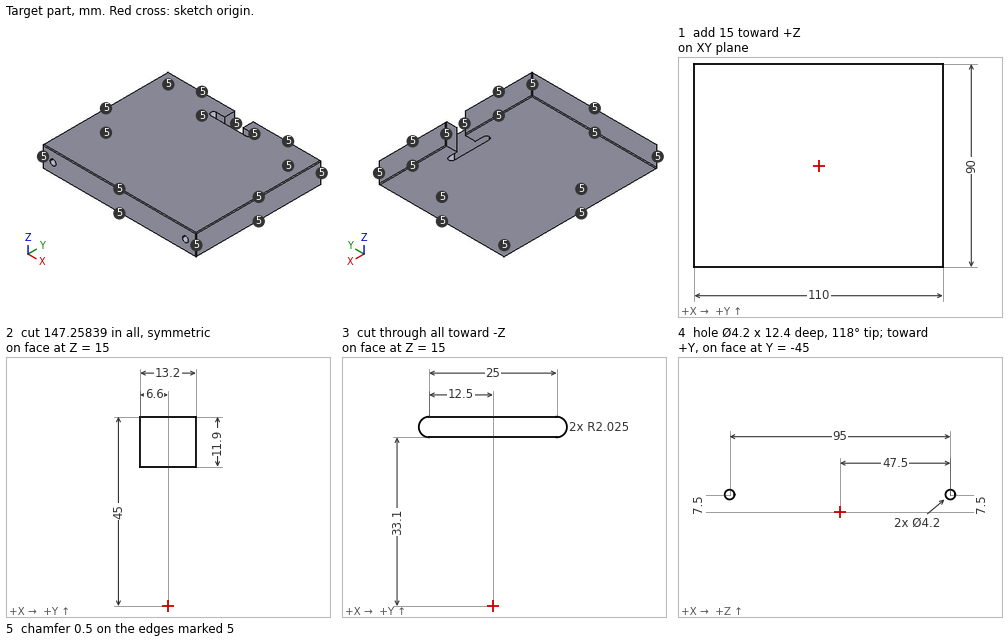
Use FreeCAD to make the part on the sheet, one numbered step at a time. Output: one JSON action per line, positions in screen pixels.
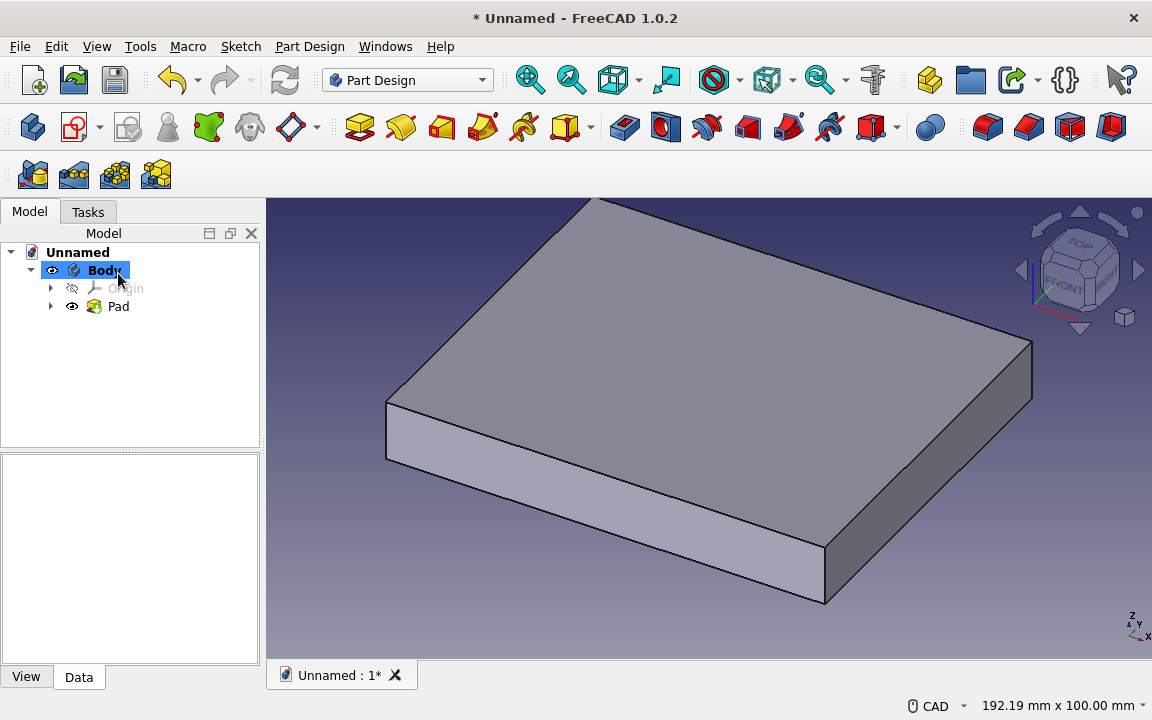
{"action": "left_click", "coordinate": [531, 80]}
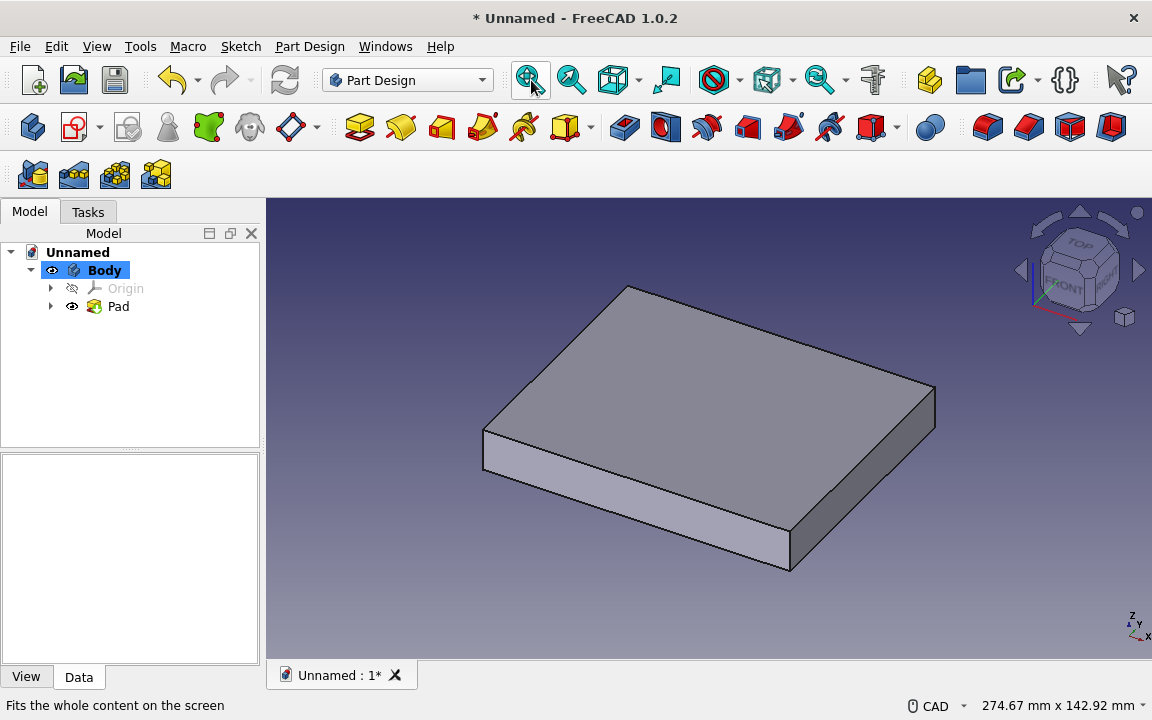
{"action": "left_click", "coordinate": [709, 408]}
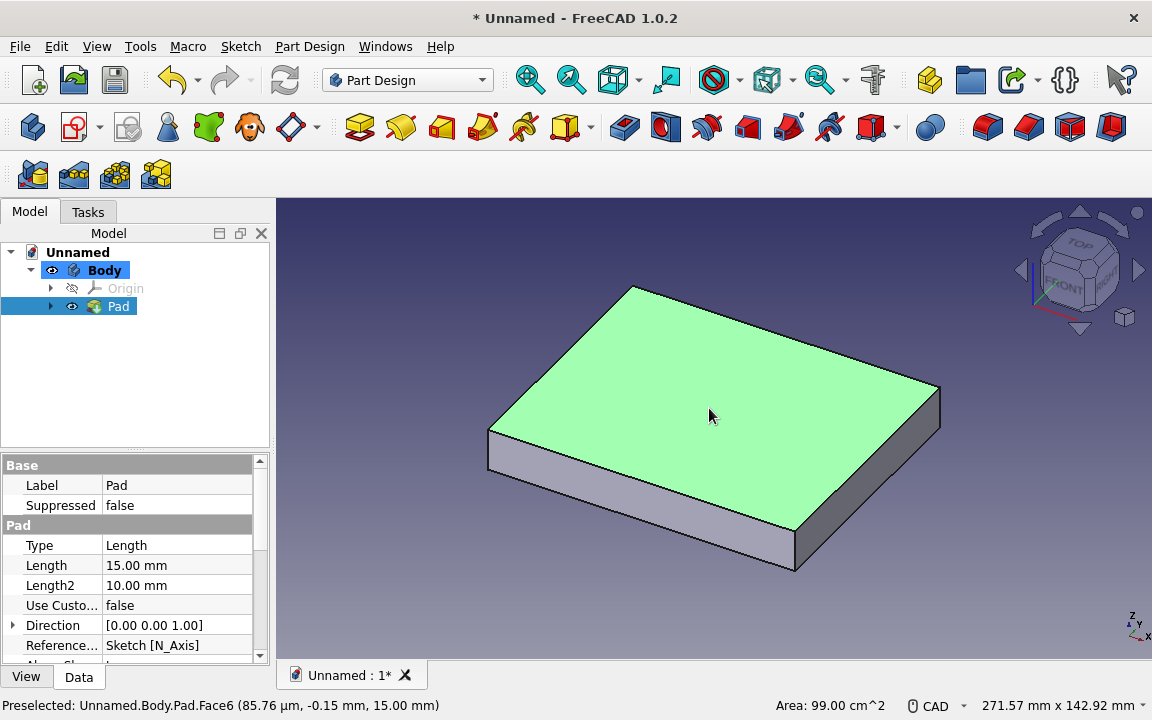
{"action": "left_click", "coordinate": [74, 128]}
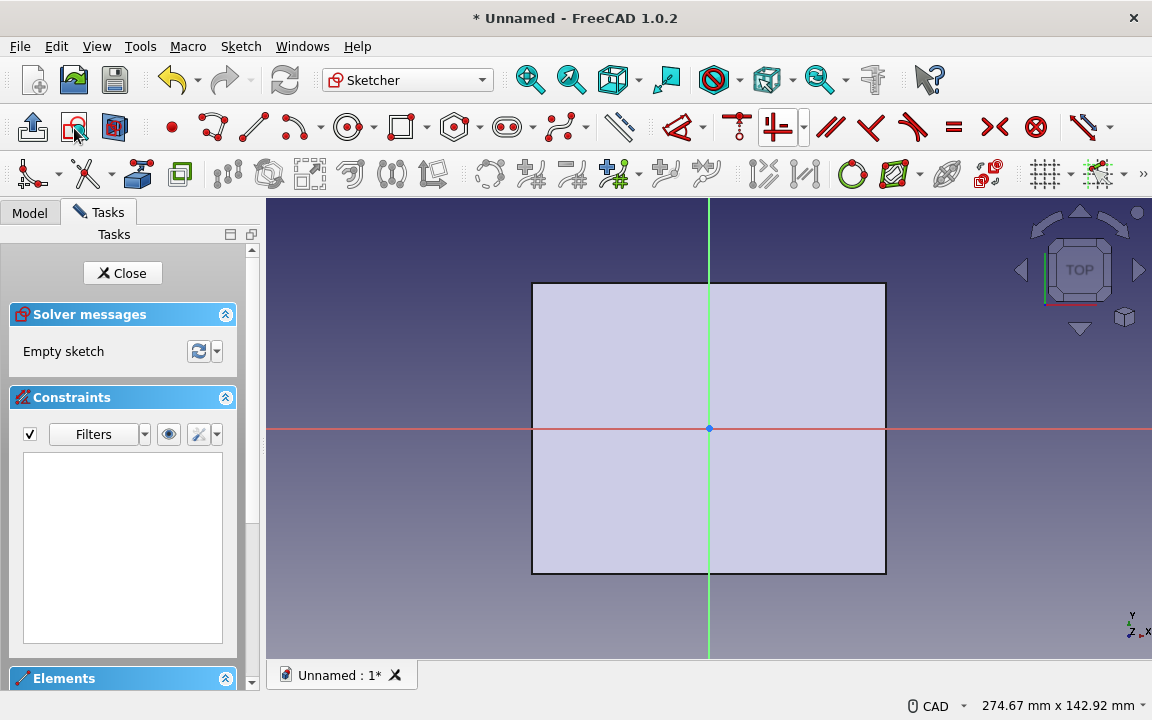
{"action": "scroll", "coordinate": [720, 283], "scroll_direction": "up", "scroll_amount": 10}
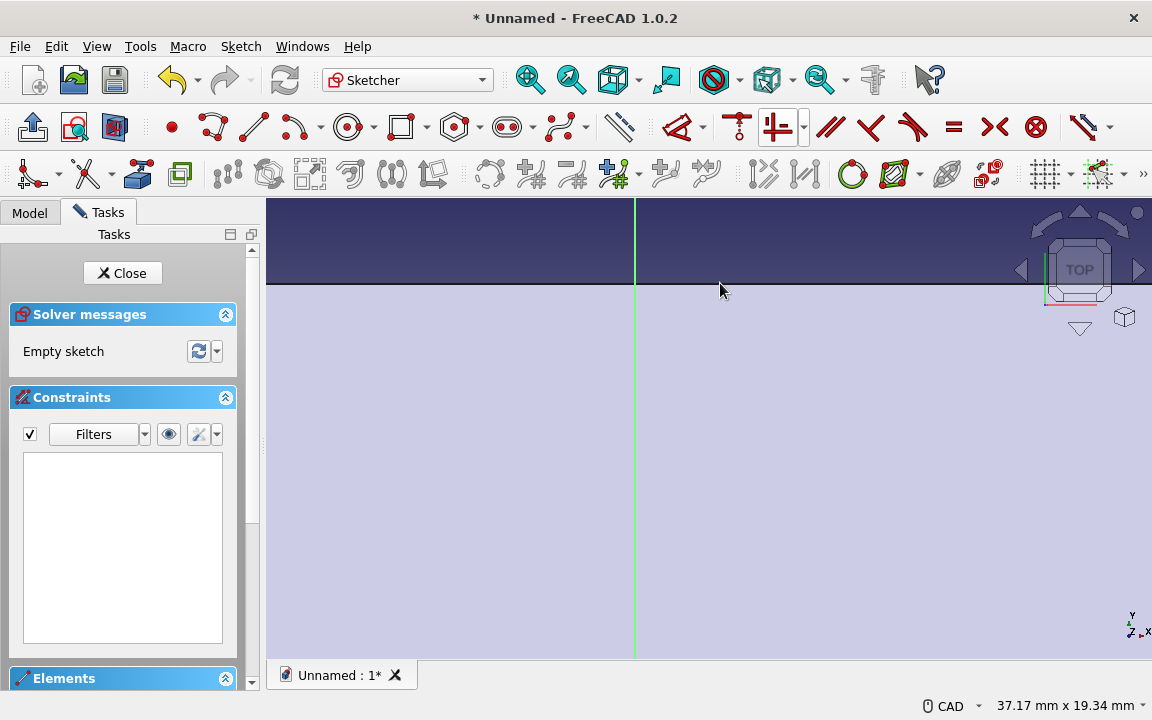
{"action": "left_click", "coordinate": [400, 128]}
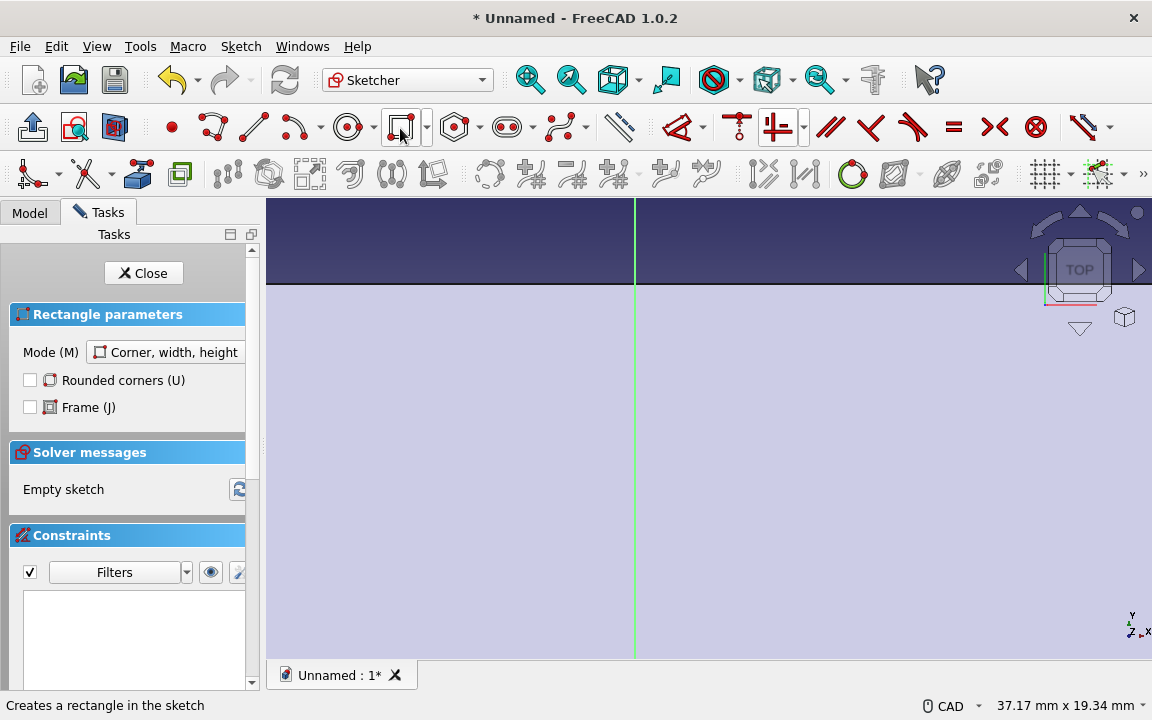
{"action": "left_click", "coordinate": [478, 284]}
{"action": "mouse_move", "coordinate": [793, 568]}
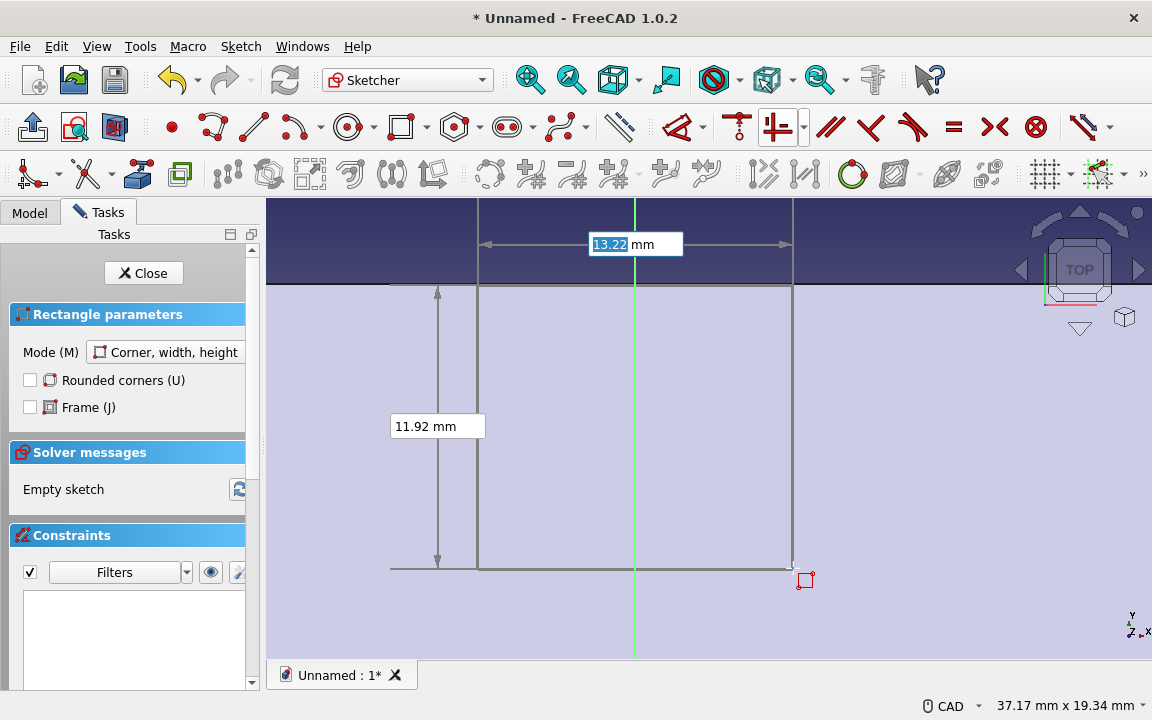
{"action": "type", "text": "13.2"}
{"action": "key", "text": "Tab"}
{"action": "type", "text": "11.9"}
{"action": "key", "text": "Return"}
{"action": "key", "text": "Escape"}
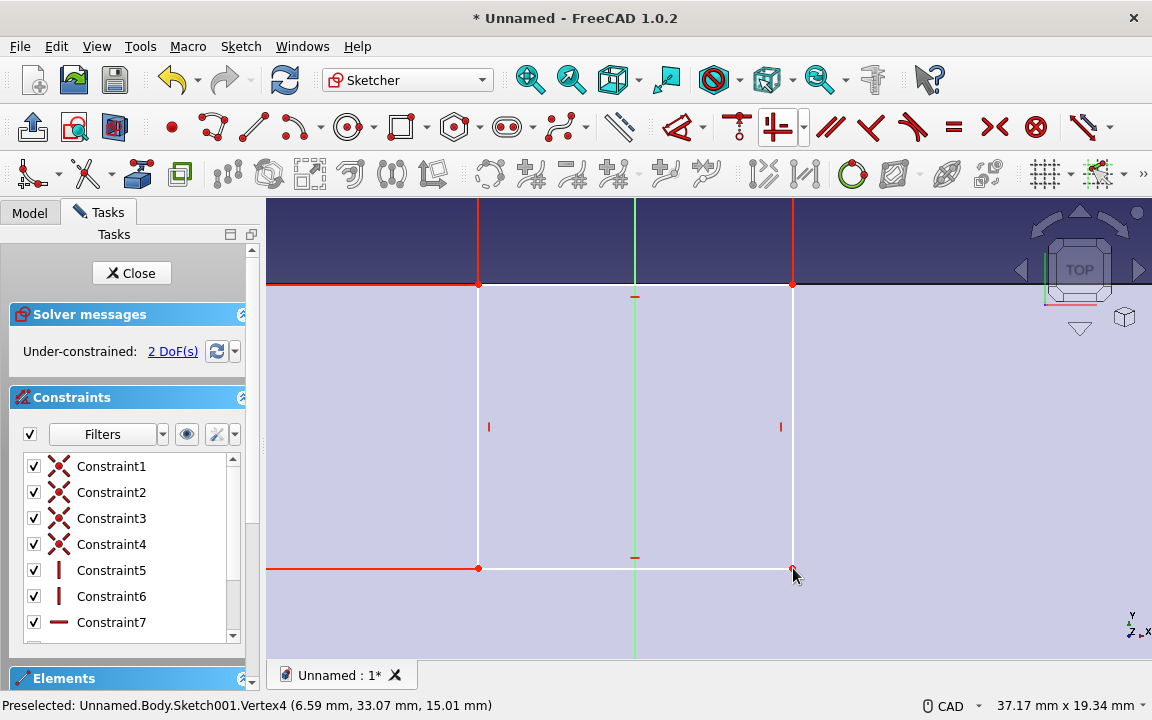
{"action": "left_click", "coordinate": [676, 128]}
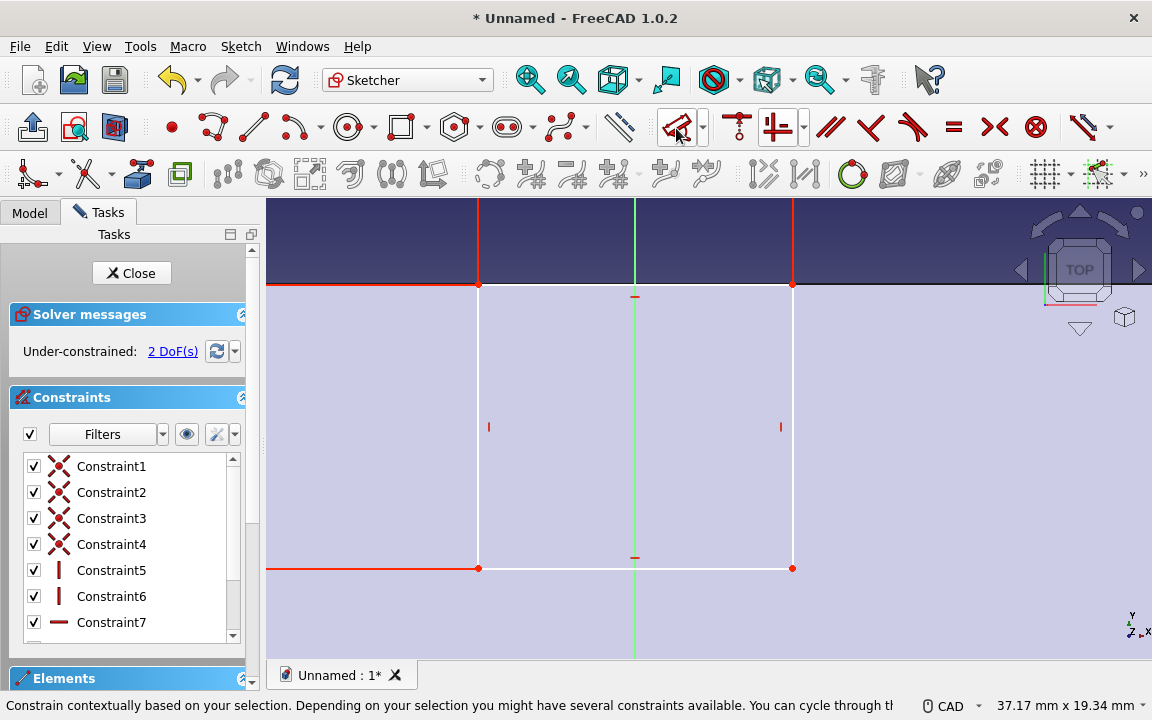
{"action": "left_click", "coordinate": [478, 285]}
{"action": "left_click", "coordinate": [444, 458]}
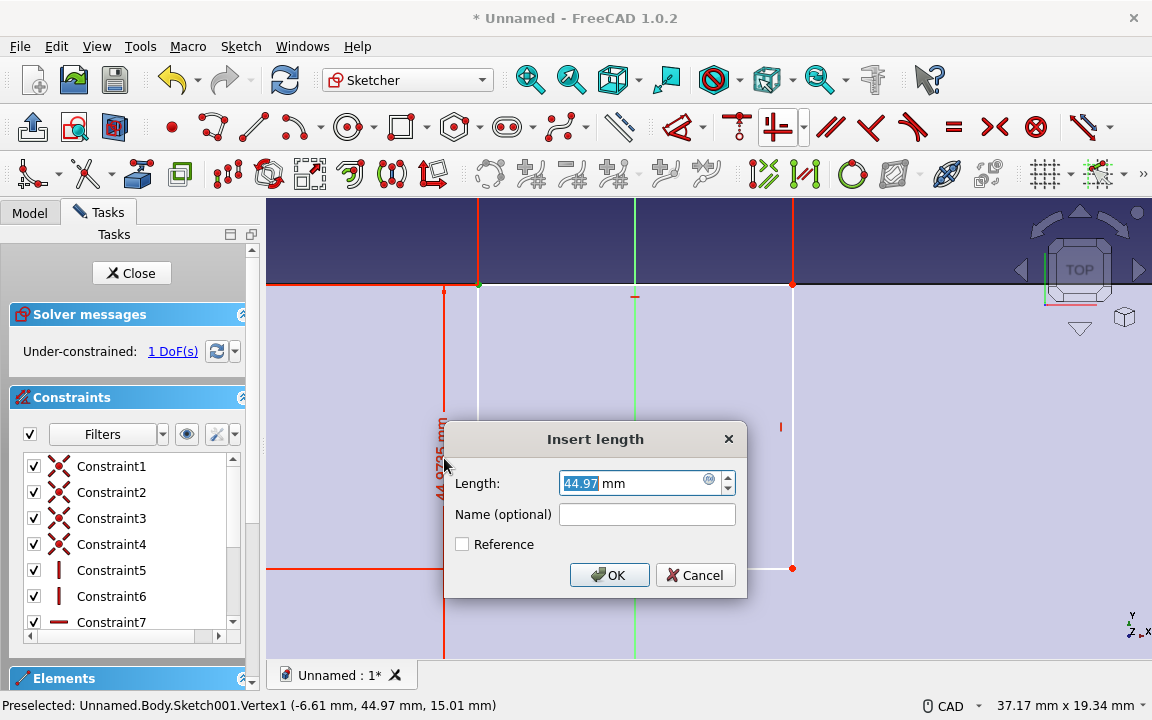
{"action": "type", "text": "45"}
{"action": "key", "text": "Return"}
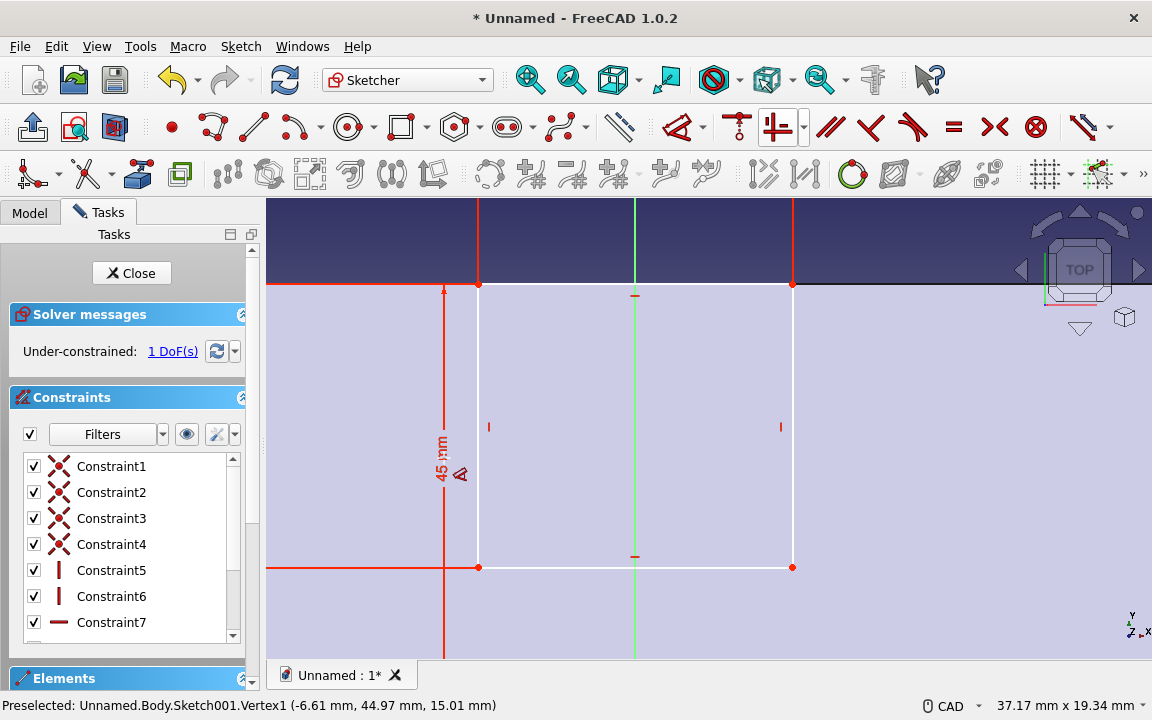
{"action": "left_click", "coordinate": [478, 284]}
{"action": "left_click", "coordinate": [557, 250]}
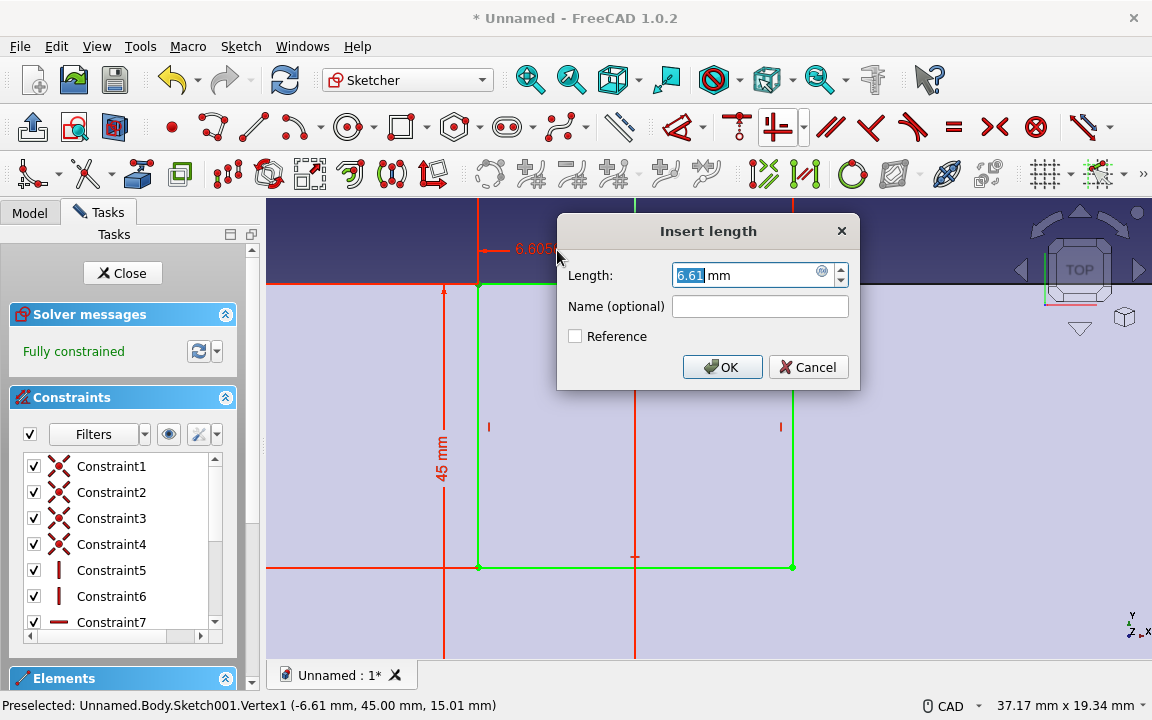
{"action": "type", "text": "6.6"}
{"action": "key", "text": "Return"}
{"action": "key", "text": "Escape"}